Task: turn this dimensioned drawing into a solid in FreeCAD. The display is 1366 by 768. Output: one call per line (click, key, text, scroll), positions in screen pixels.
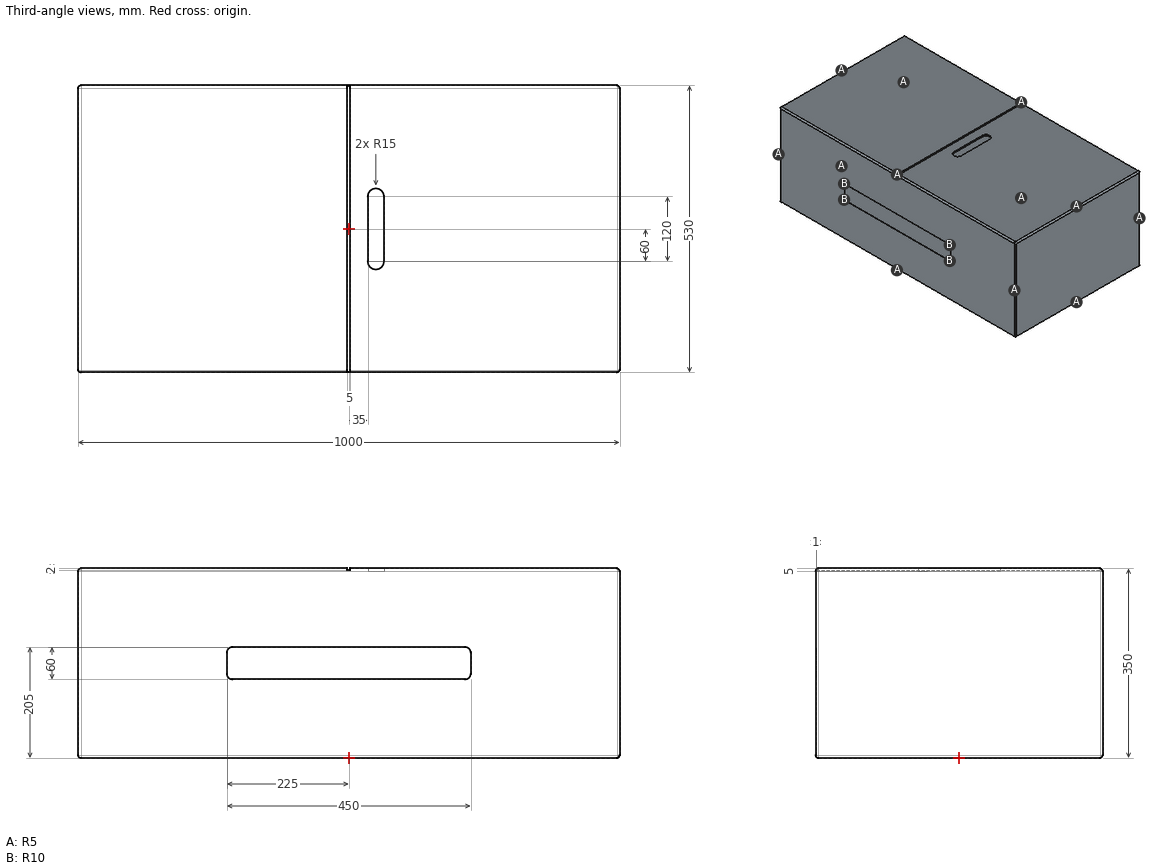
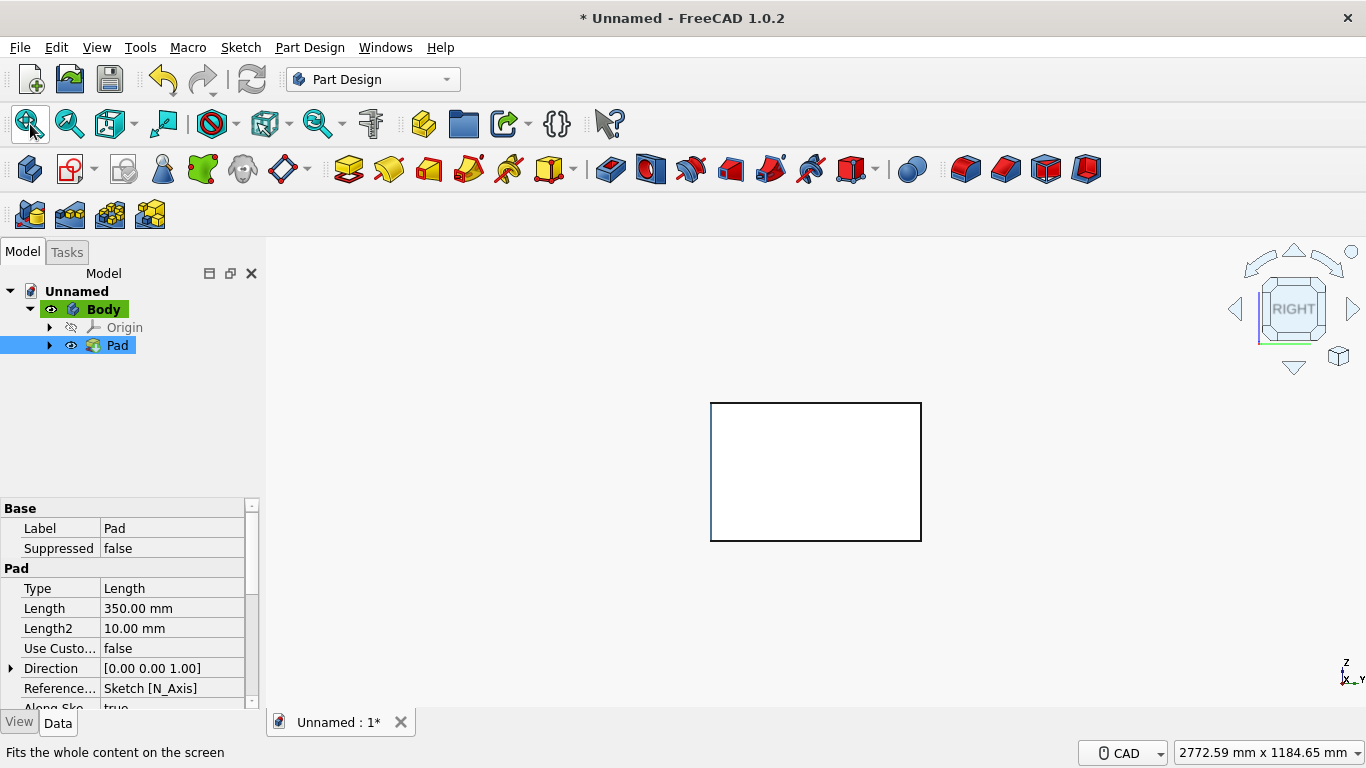
click(921, 471, ctrl)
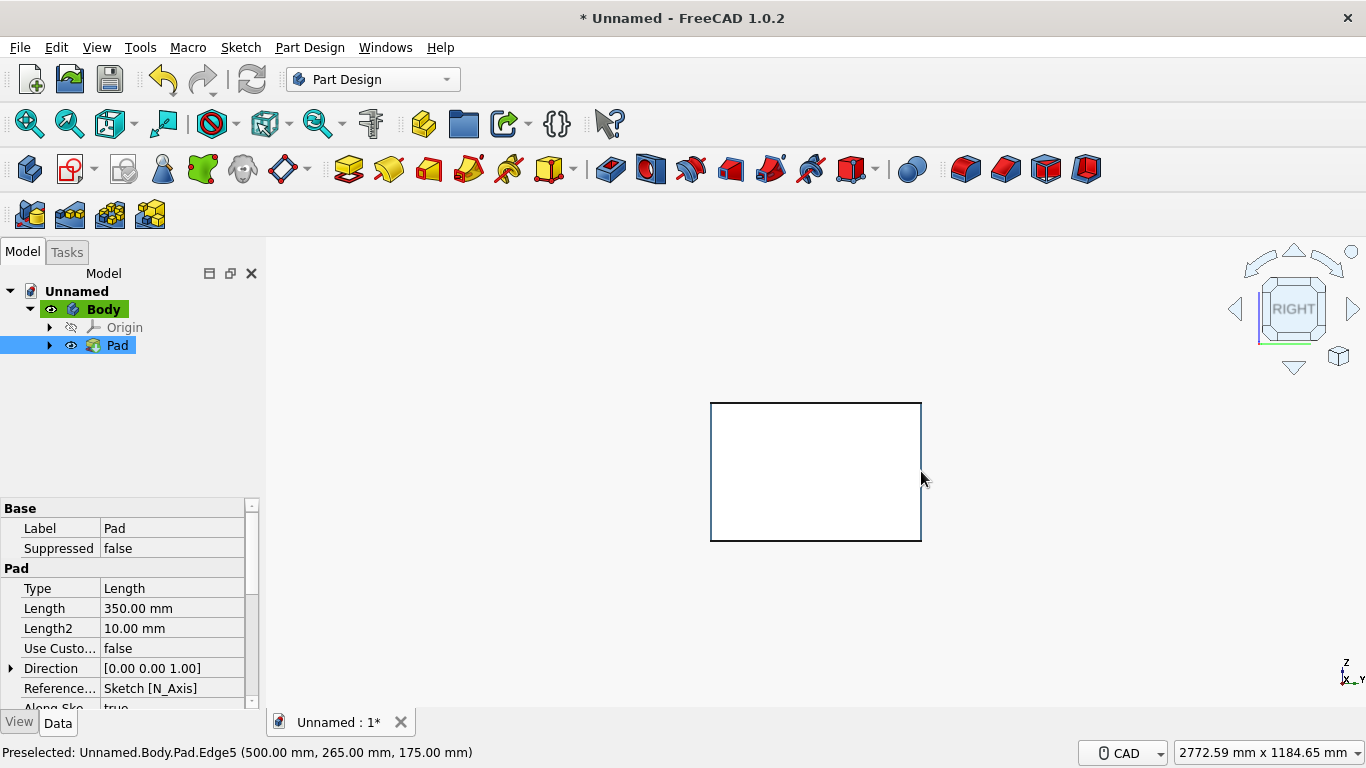
key(5)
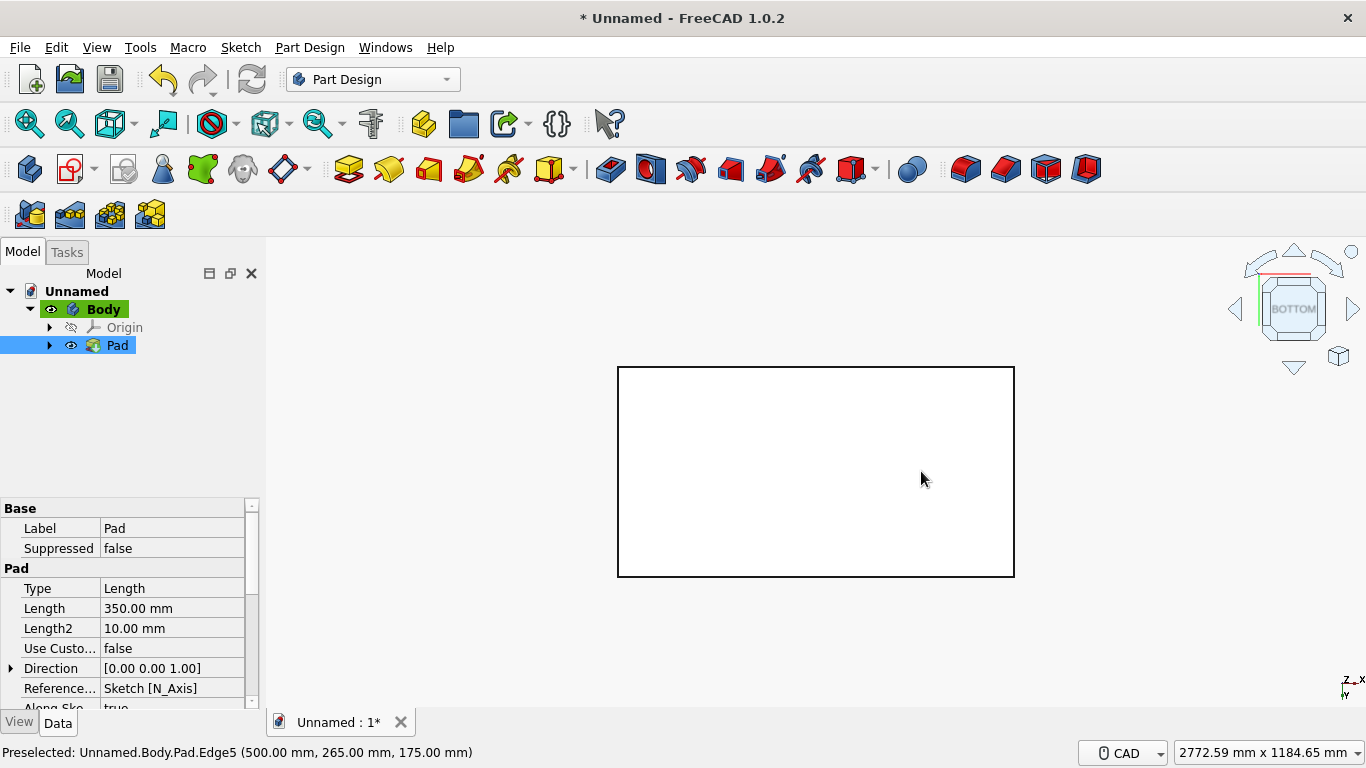
click(30, 124)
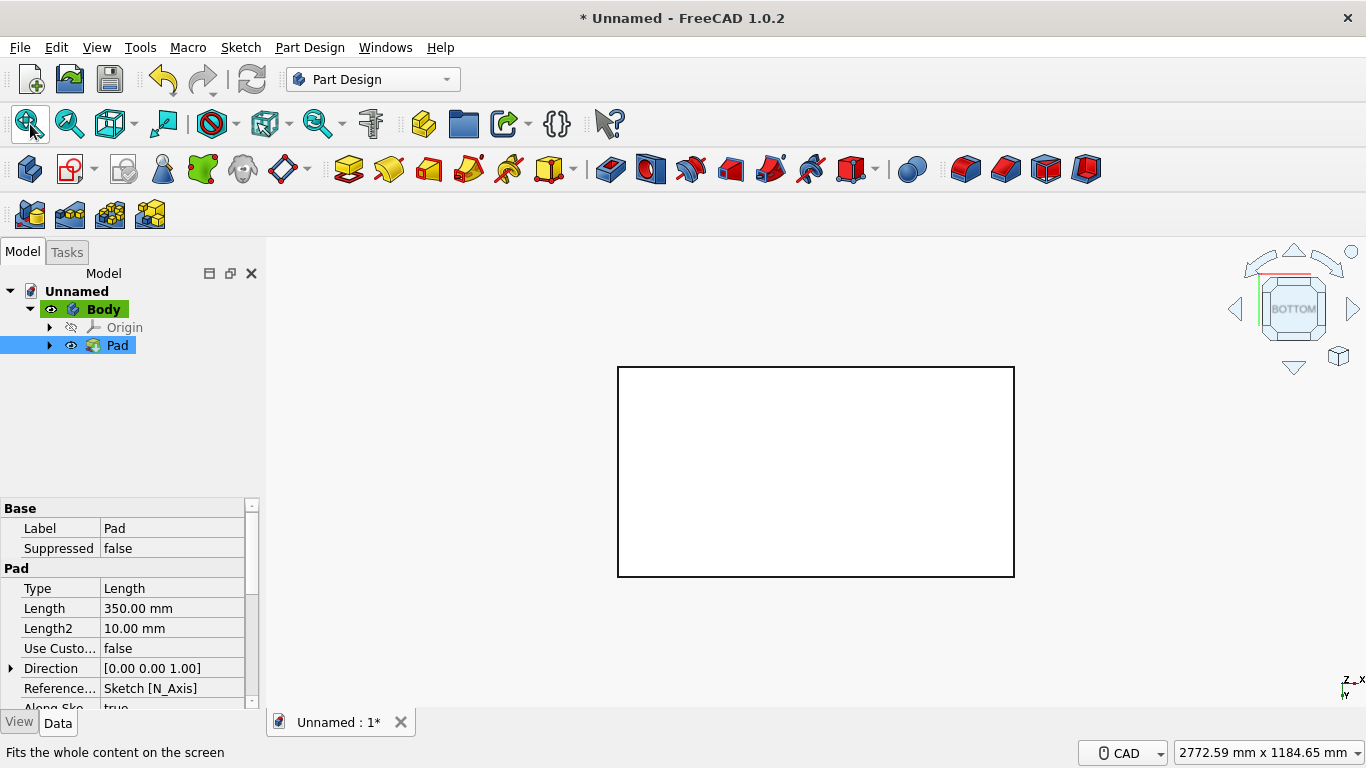
click(873, 471, ctrl)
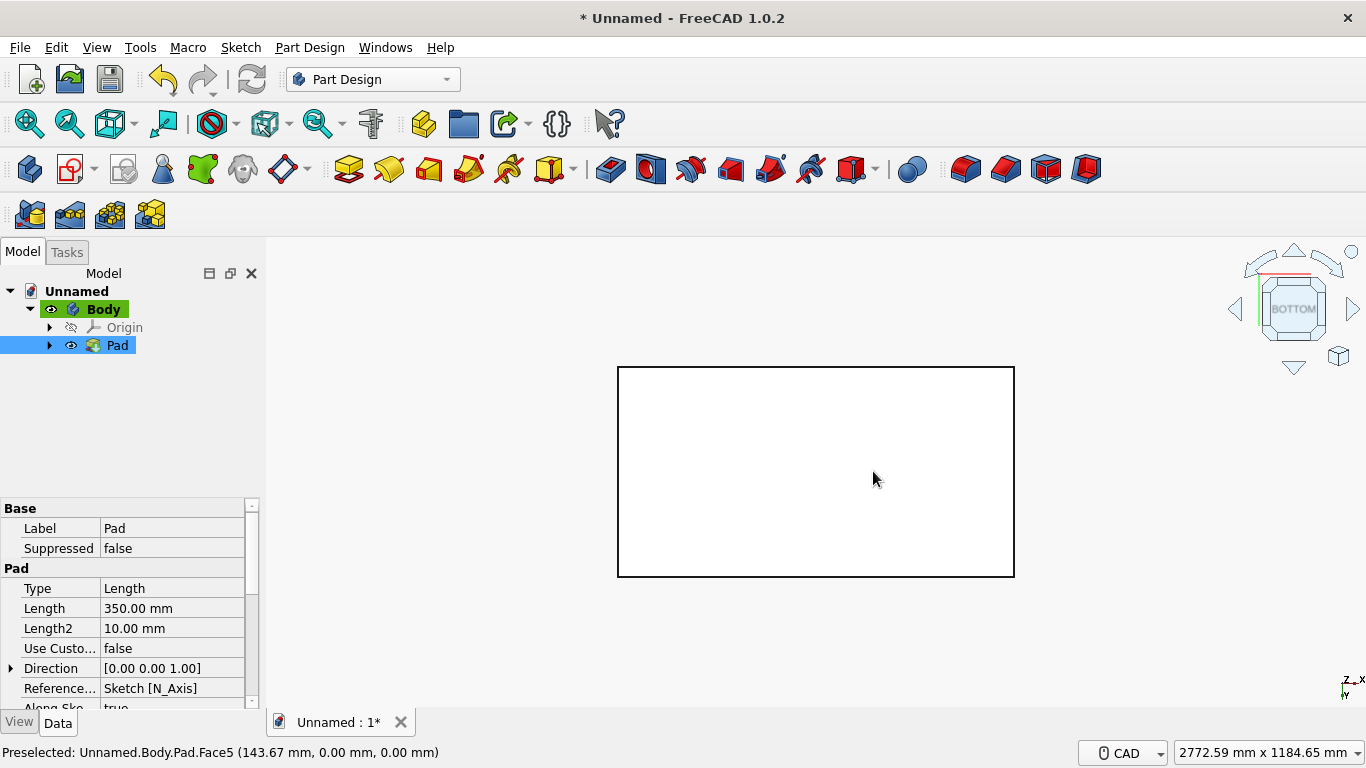
key(4)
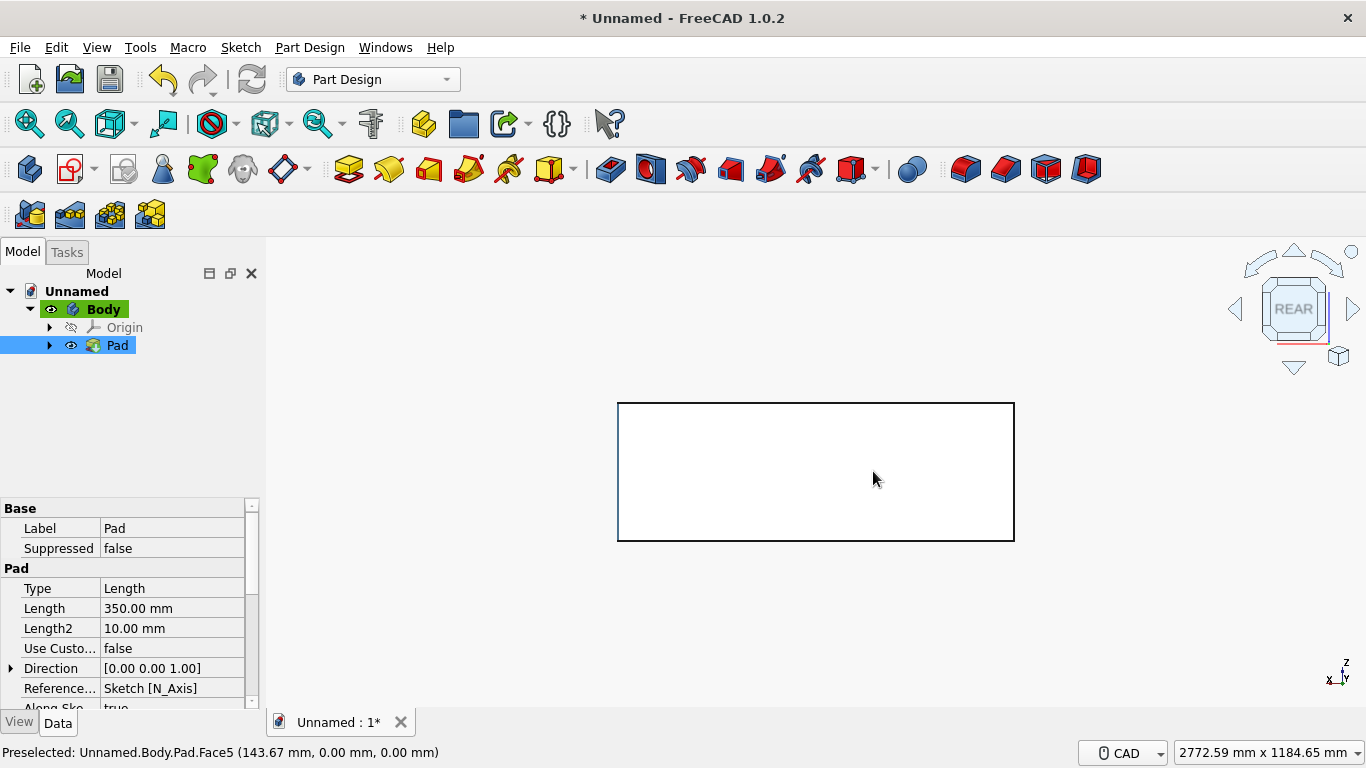
click(30, 124)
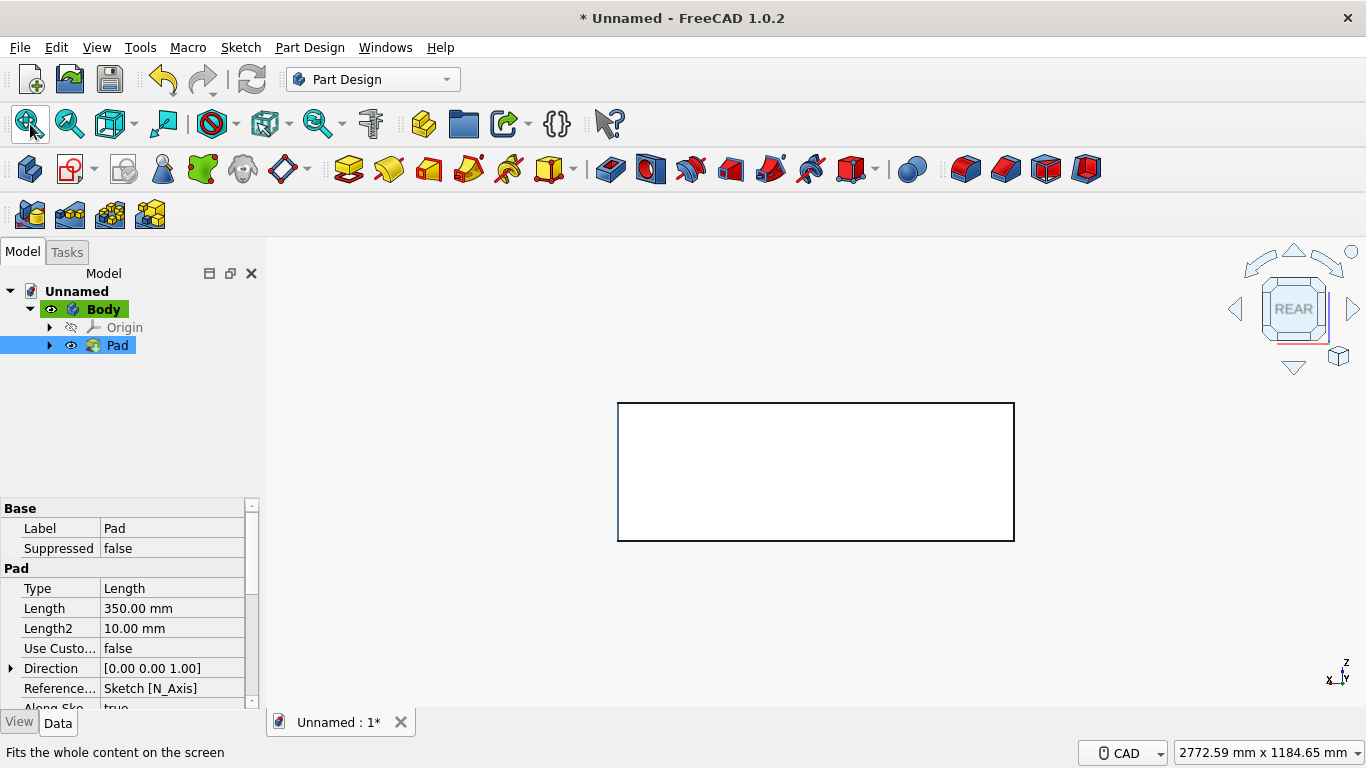
click(1014, 471, ctrl)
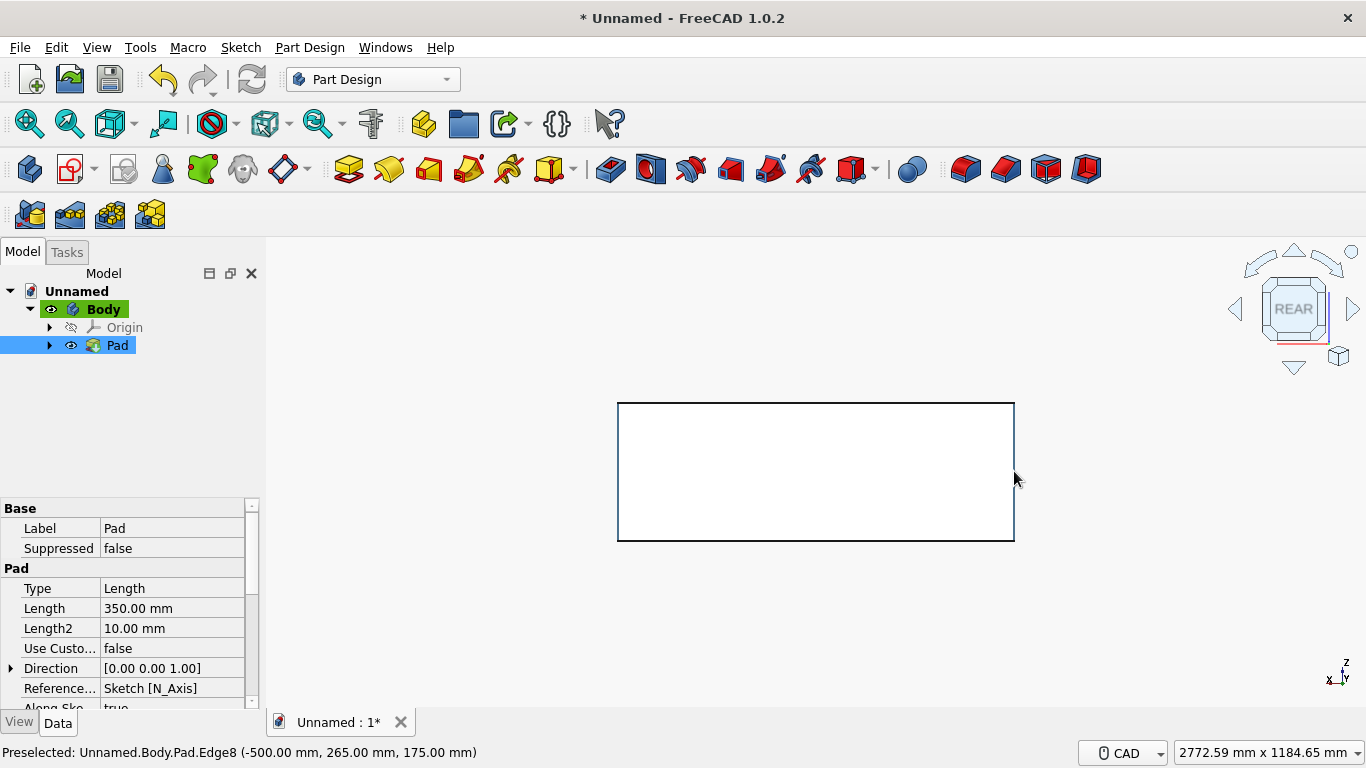
click(966, 170)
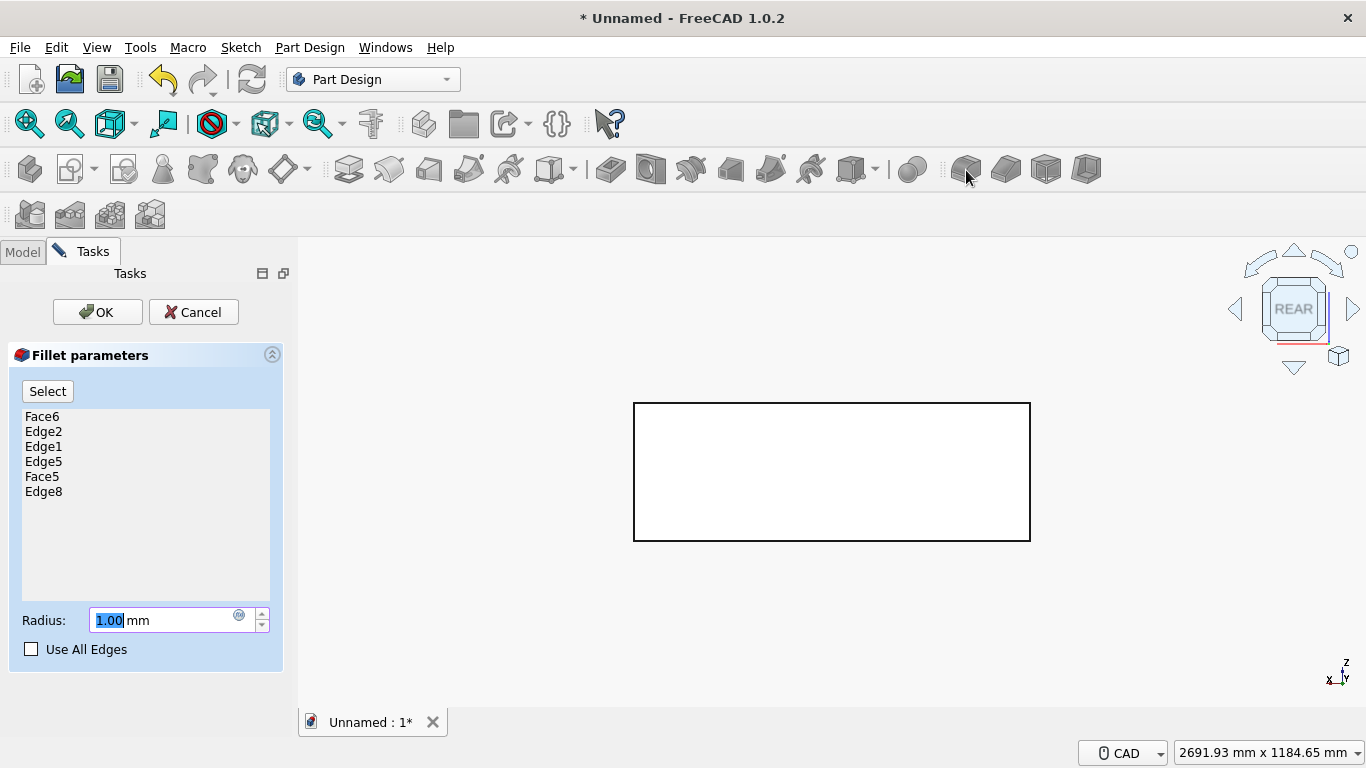
text(5)
key(Tab)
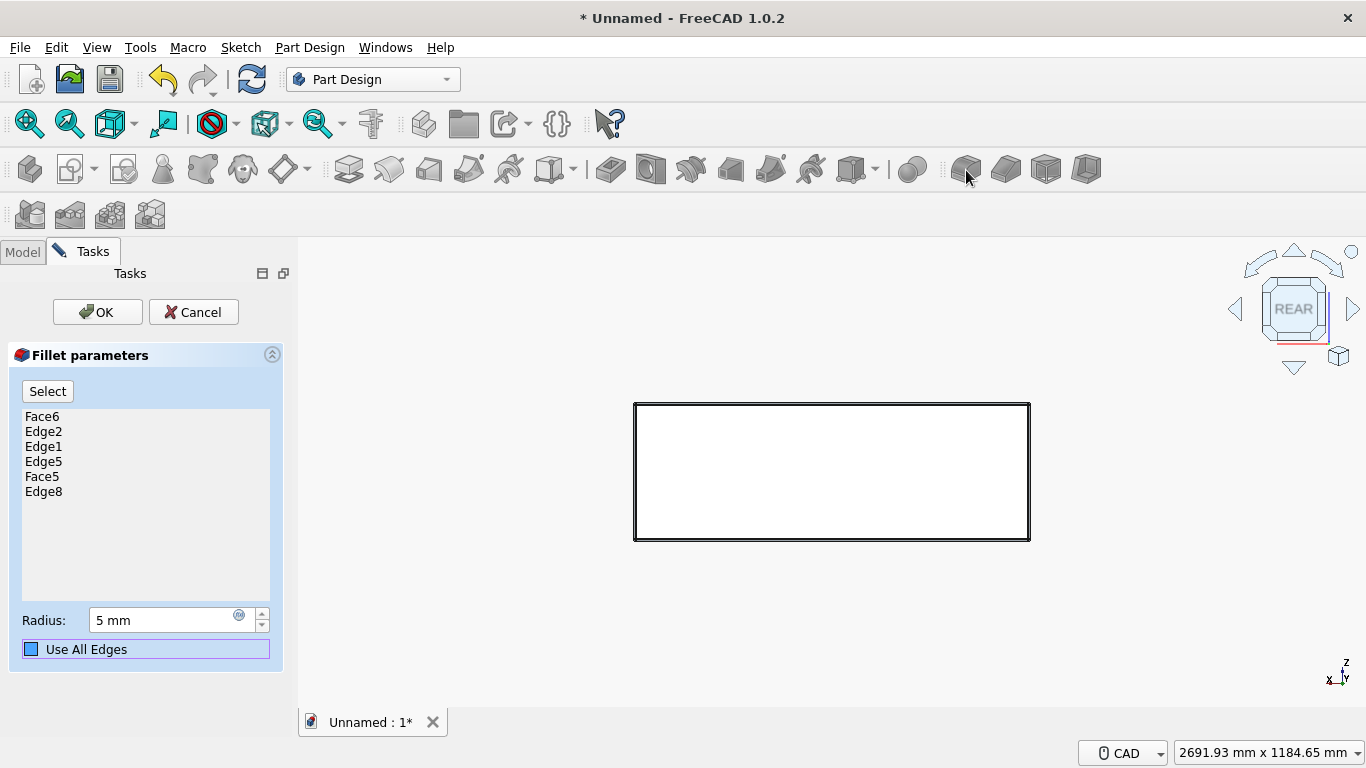
click(98, 312)